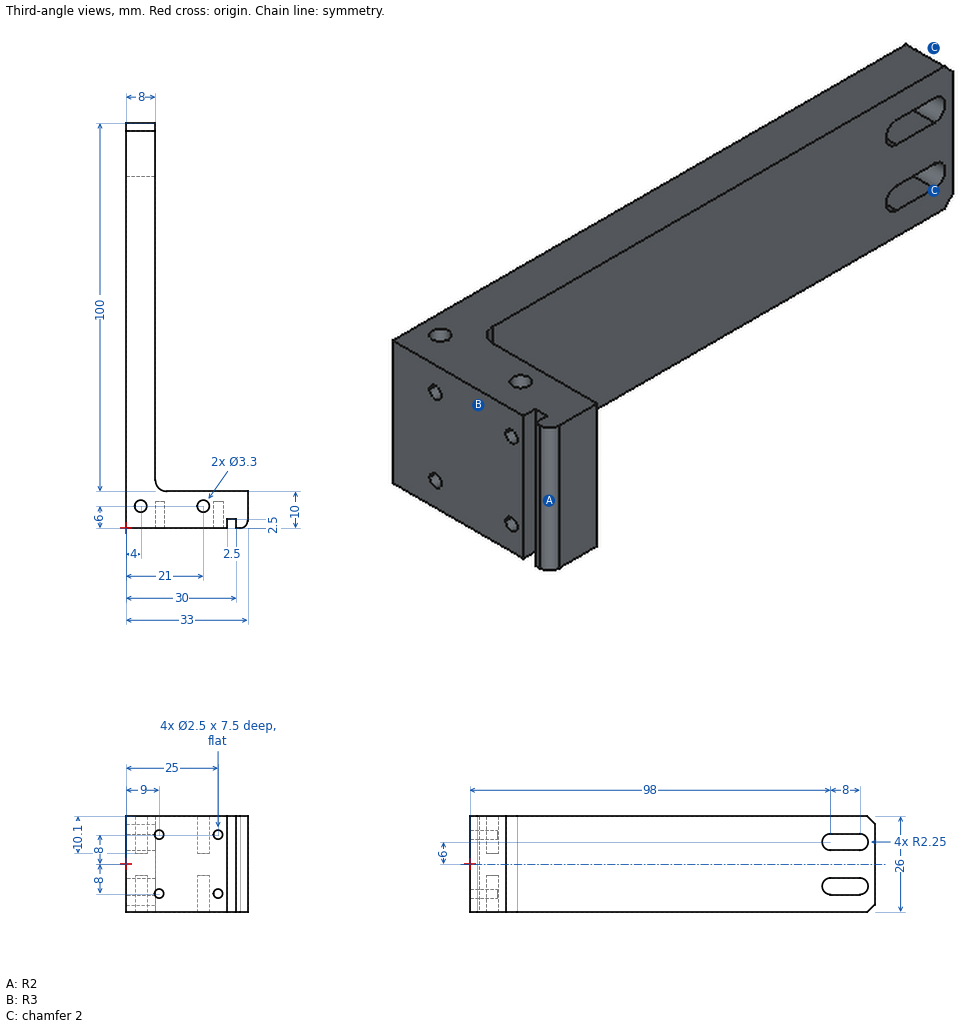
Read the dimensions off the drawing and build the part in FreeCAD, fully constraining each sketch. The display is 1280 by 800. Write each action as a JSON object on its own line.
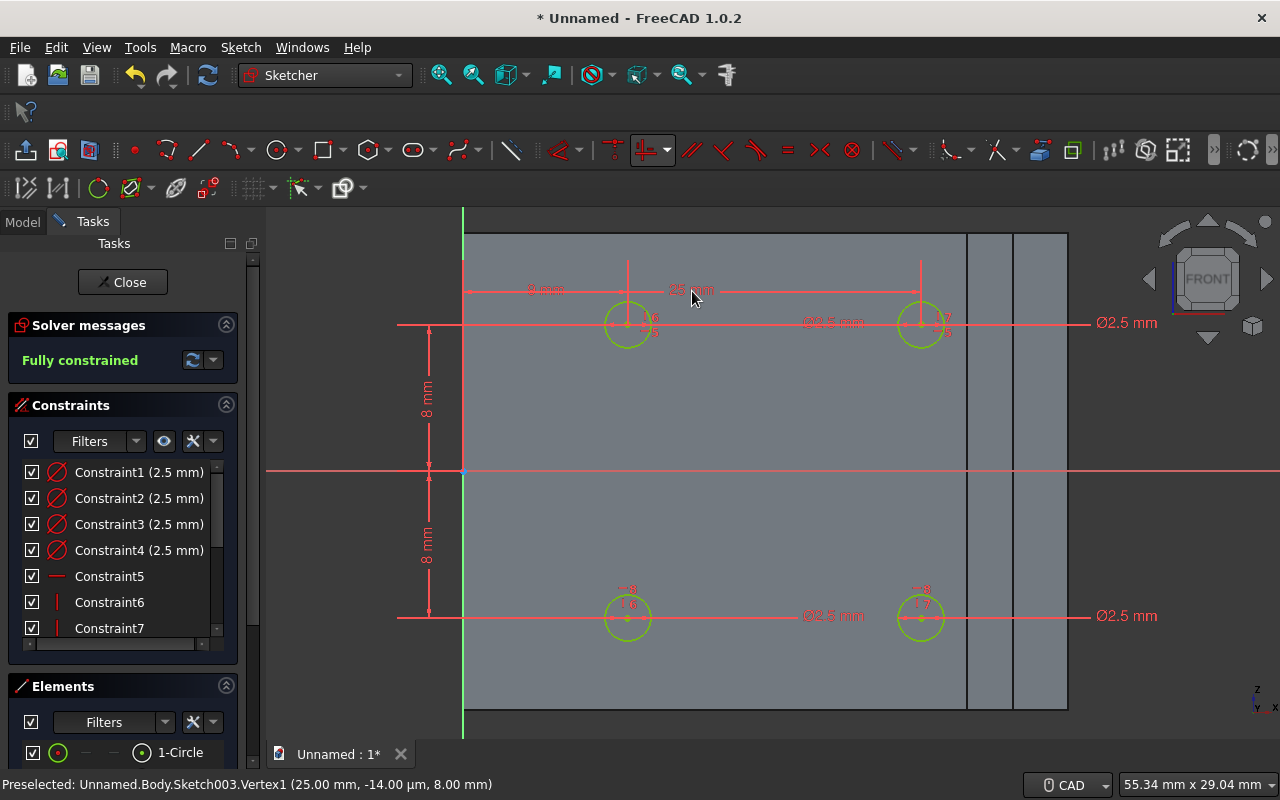
{"action": "left_click", "coordinate": [123, 282]}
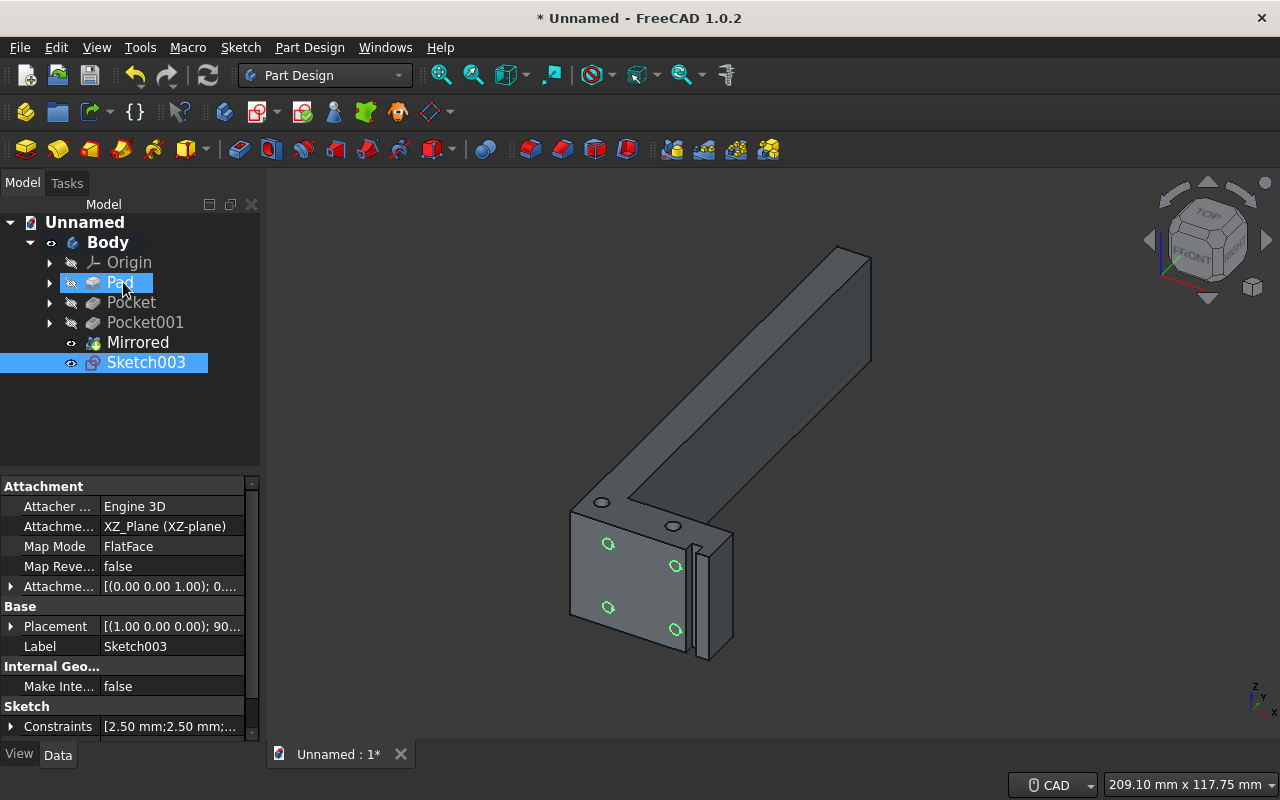
{"action": "left_click", "coordinate": [272, 150]}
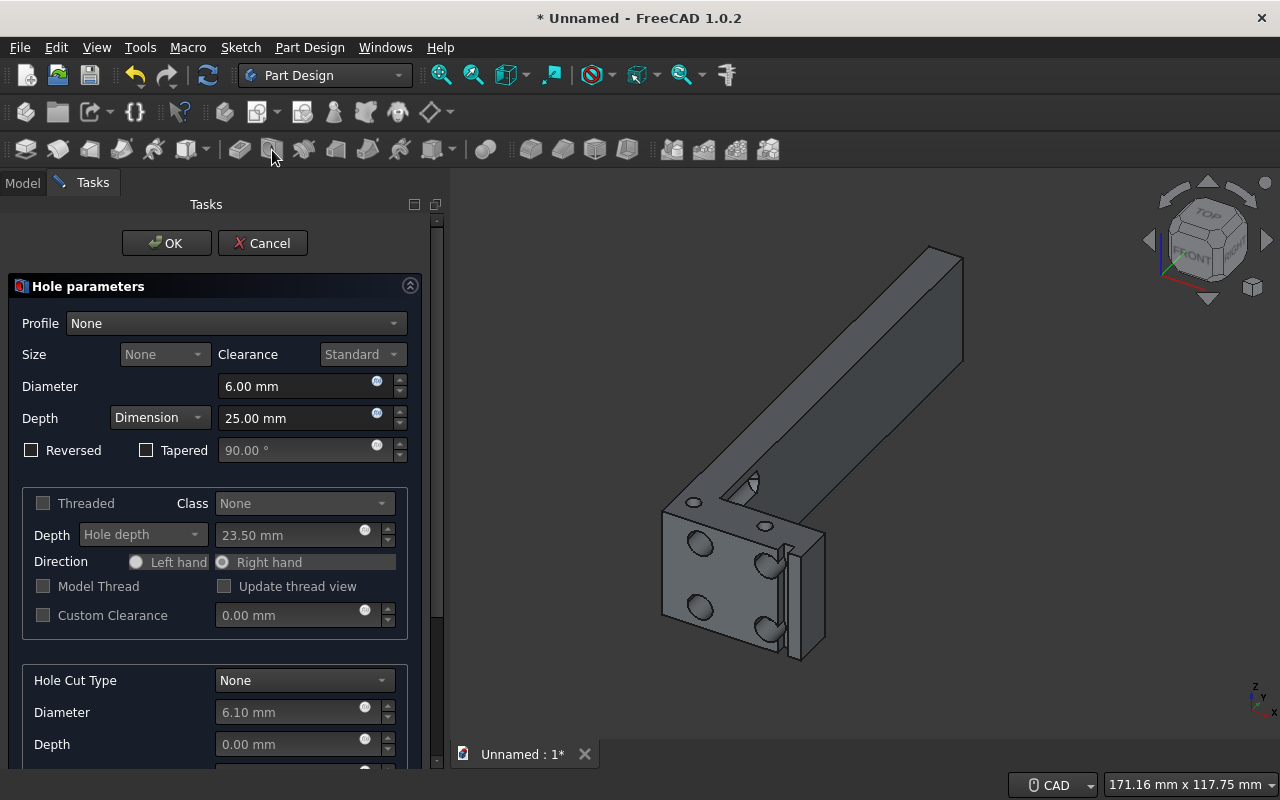
{"action": "triple_click", "coordinate": [305, 386]}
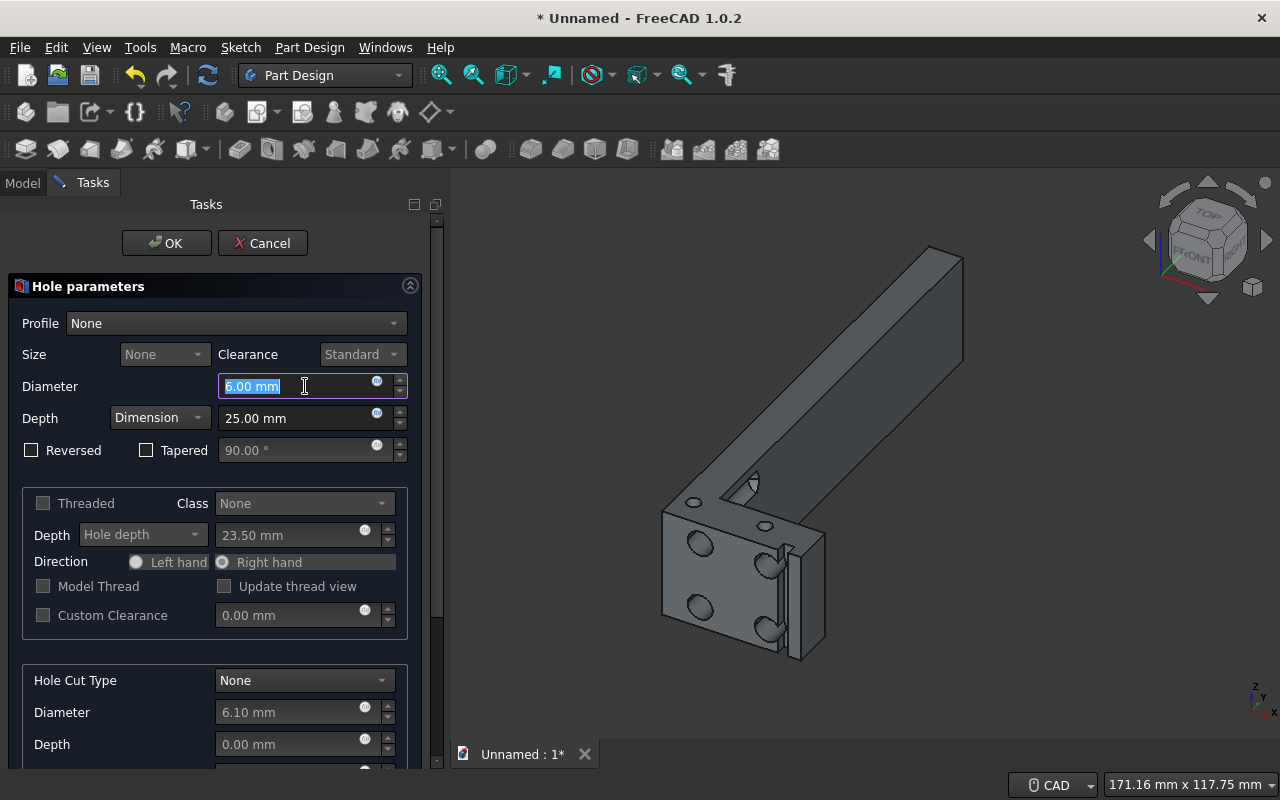
{"action": "type", "text": "2.5"}
{"action": "key", "text": "Tab"}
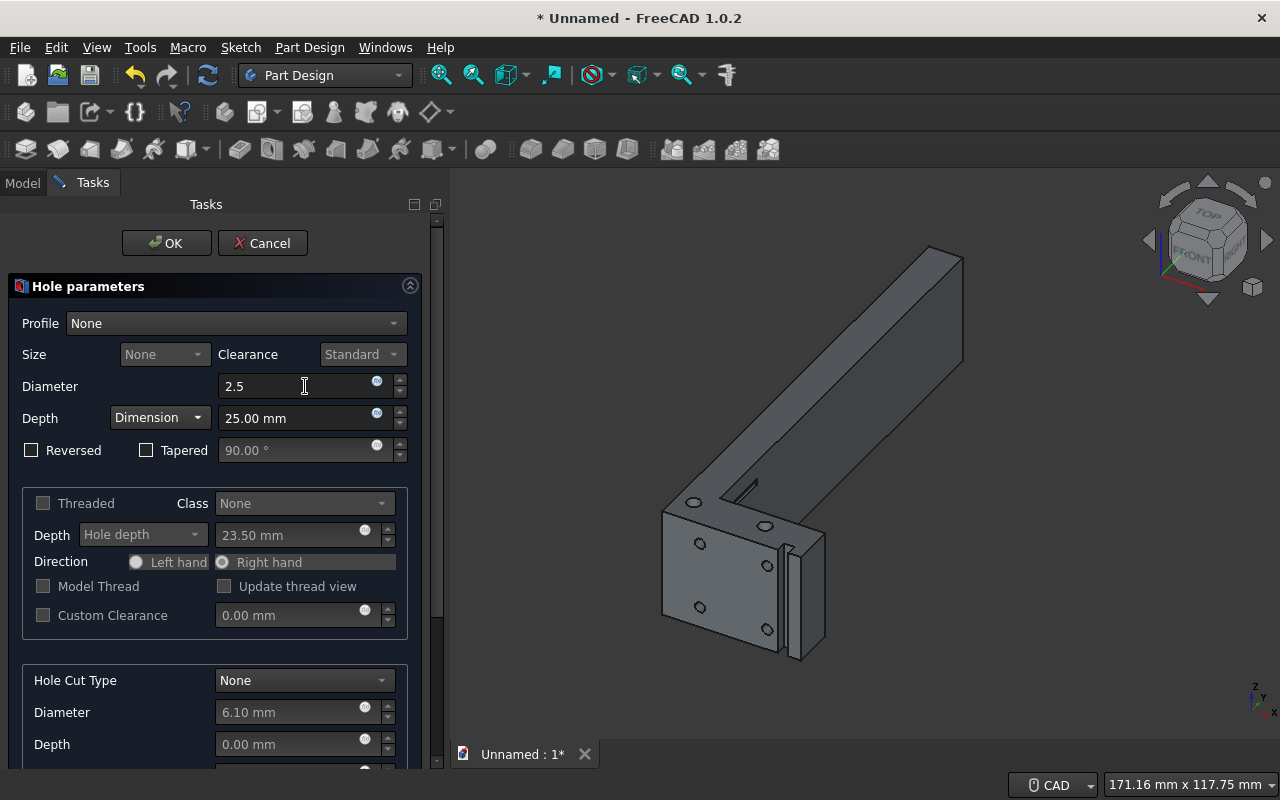
{"action": "triple_click", "coordinate": [305, 418]}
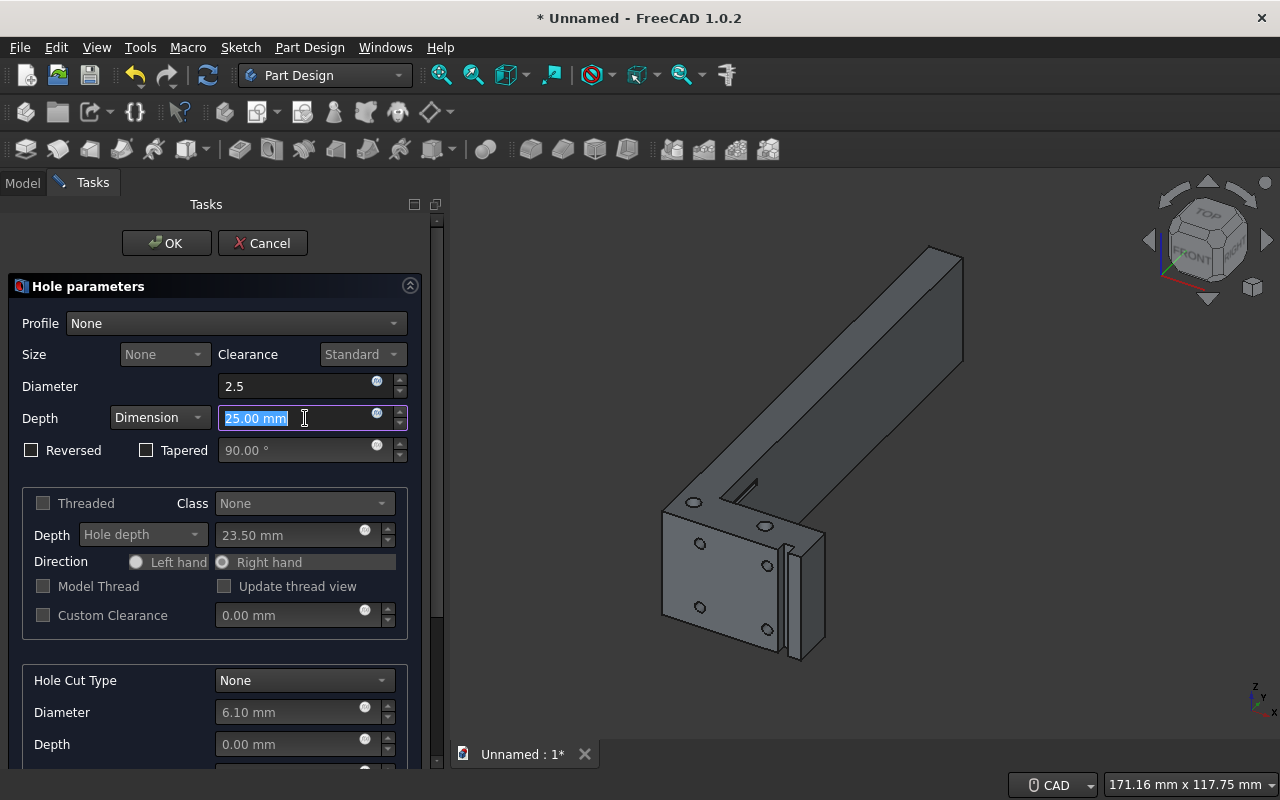
{"action": "type", "text": "7.5"}
{"action": "key", "text": "Tab"}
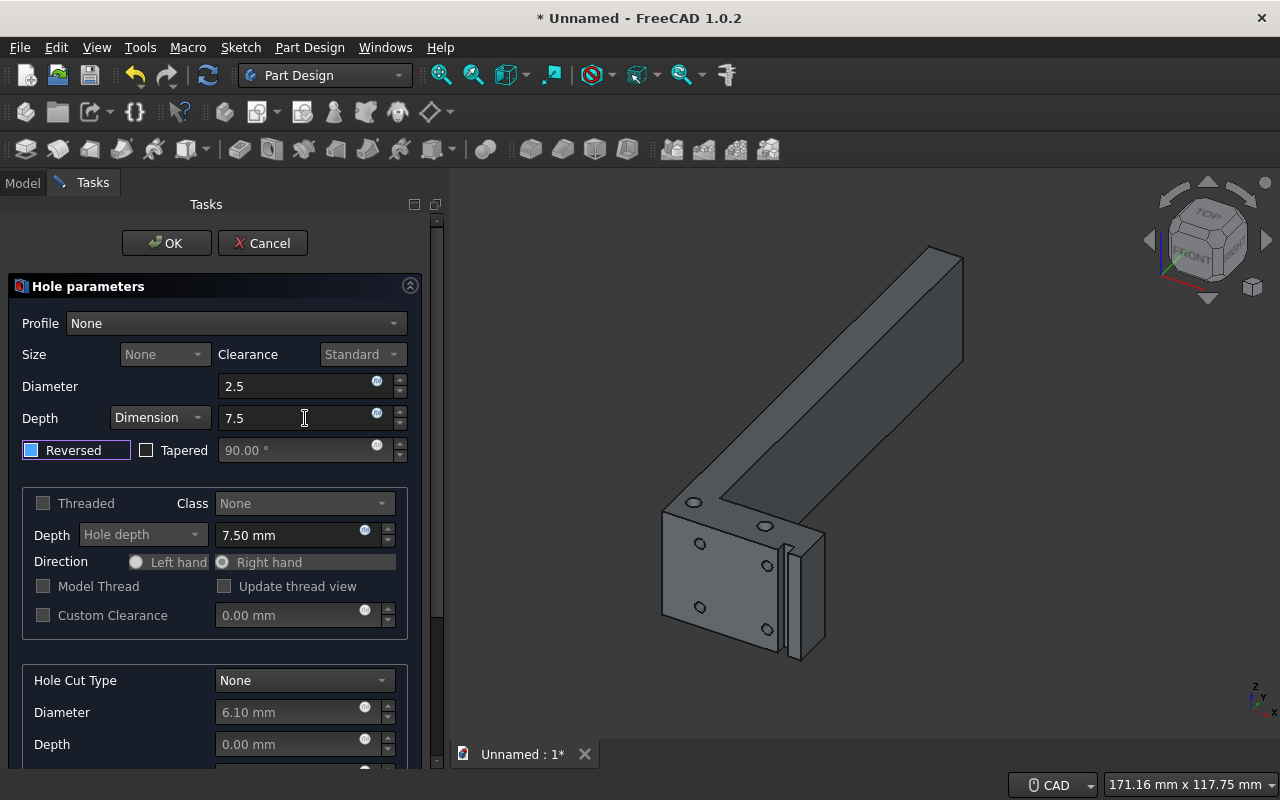
{"action": "scroll", "coordinate": [437, 491], "scroll_direction": "down", "scroll_amount": 3}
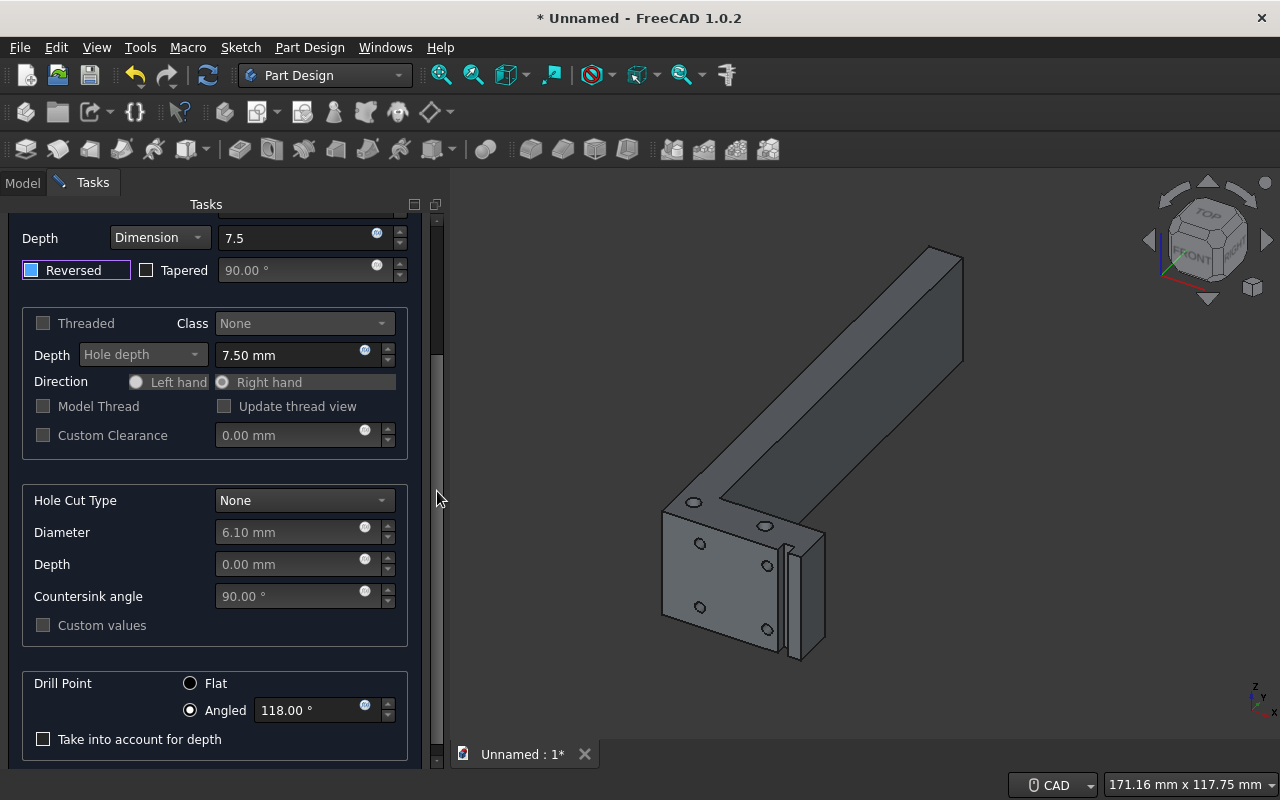
{"action": "left_click", "coordinate": [191, 683]}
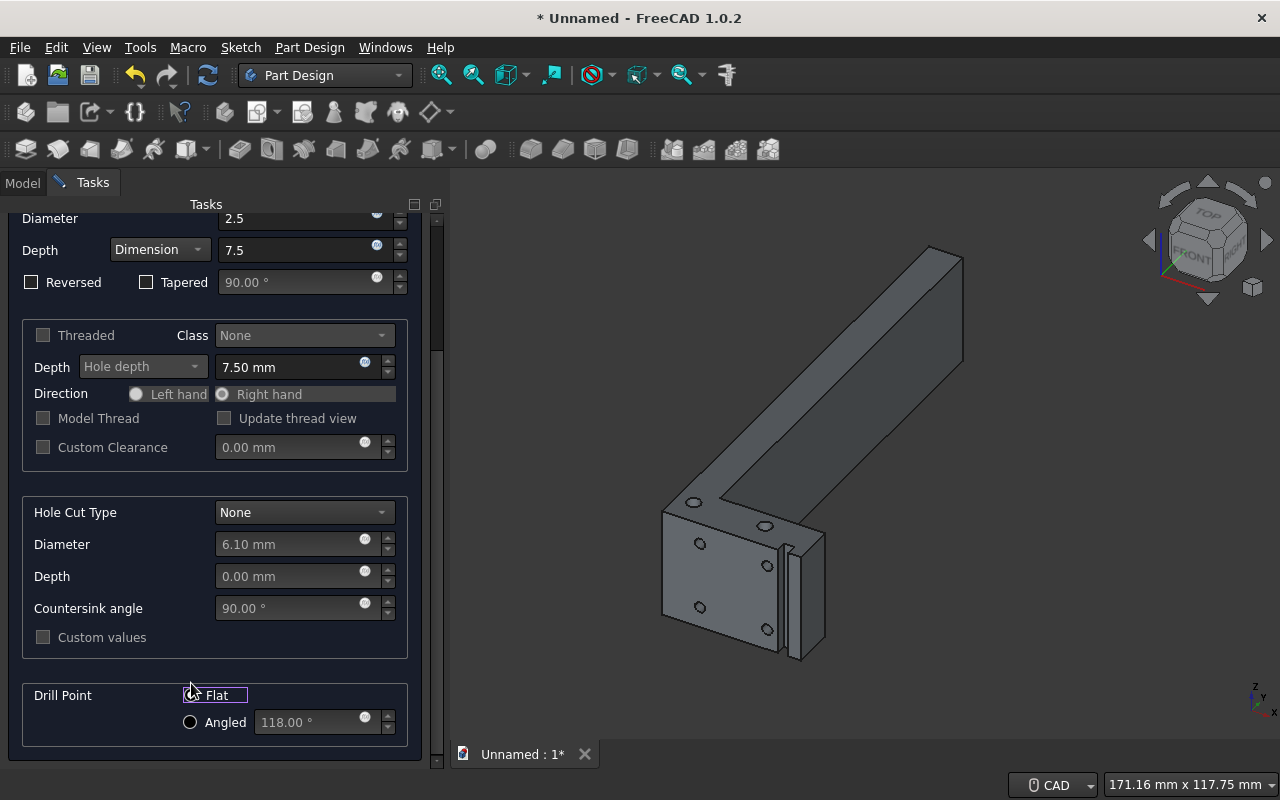
{"action": "scroll", "coordinate": [437, 491], "scroll_direction": "up", "scroll_amount": 4}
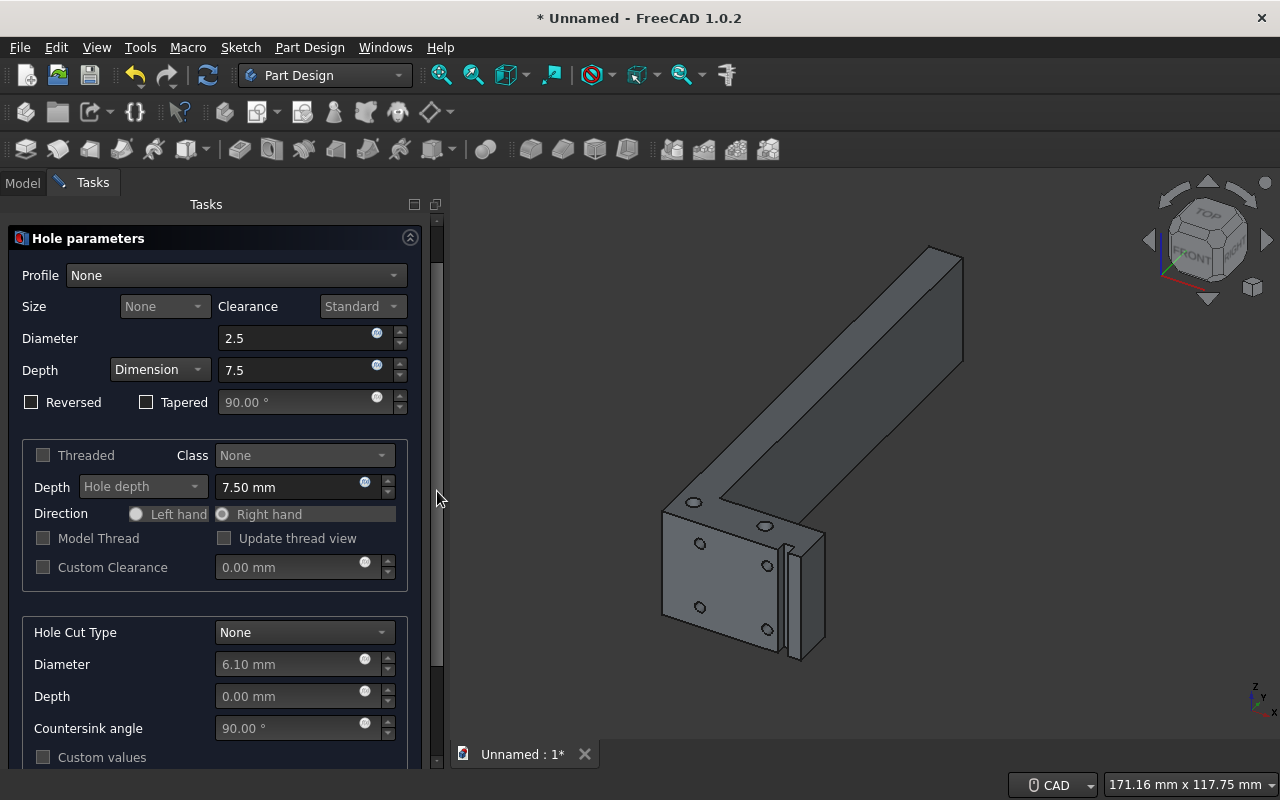
{"action": "left_click", "coordinate": [167, 243]}